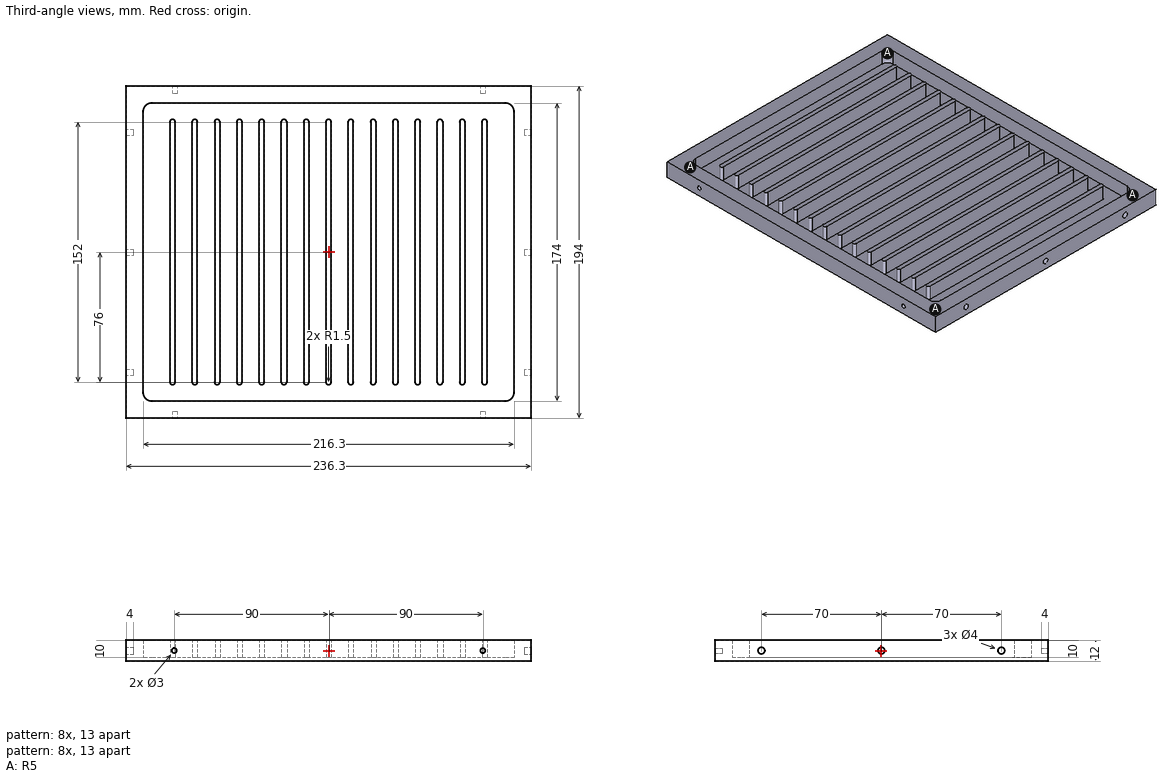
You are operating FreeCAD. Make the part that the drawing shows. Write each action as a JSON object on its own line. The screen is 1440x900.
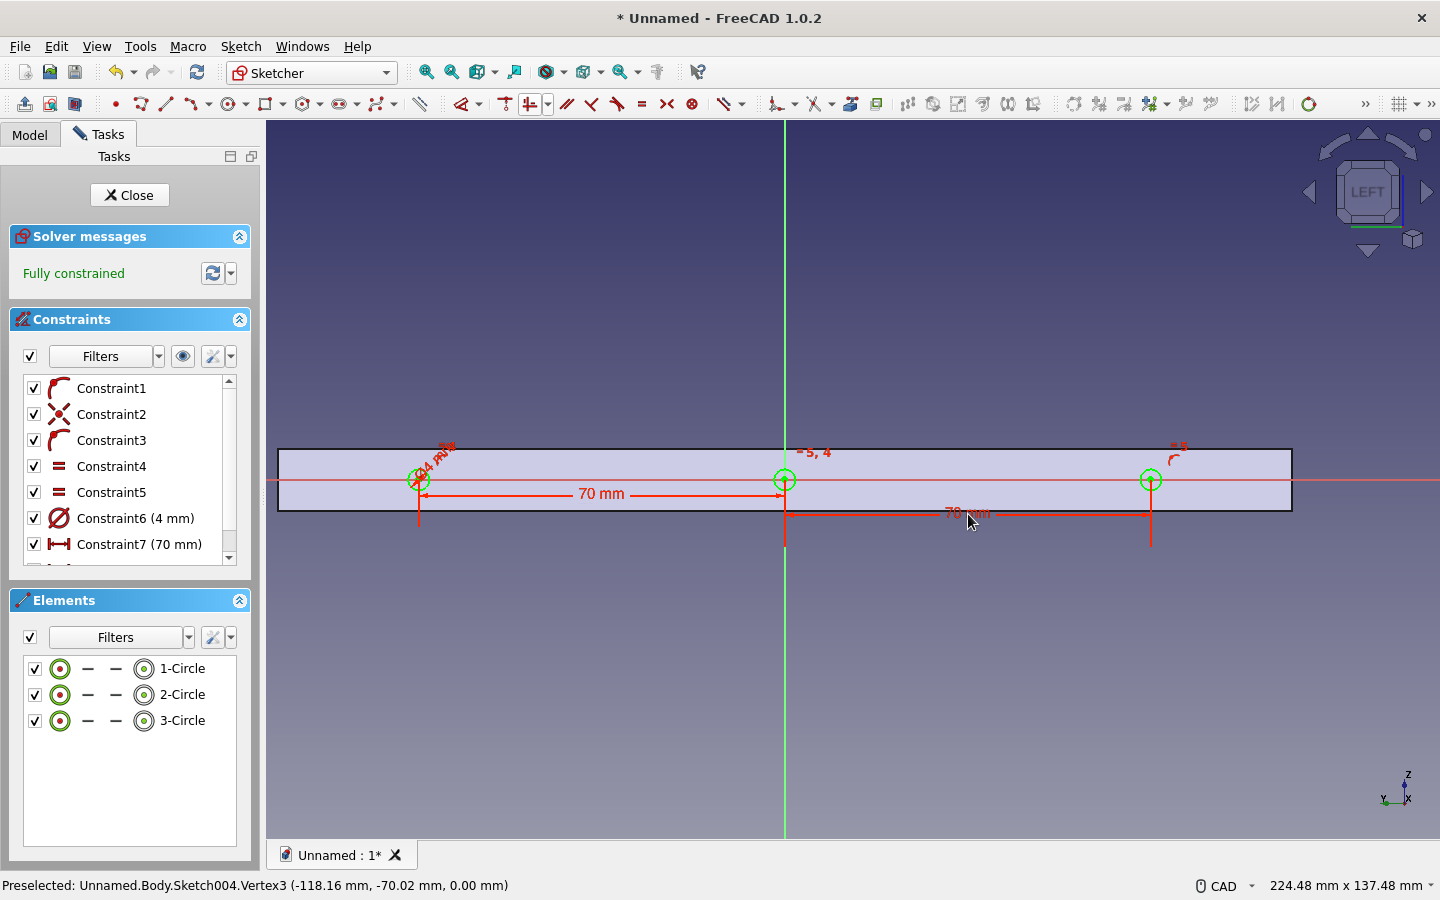
{"action": "left_click", "coordinate": [130, 195]}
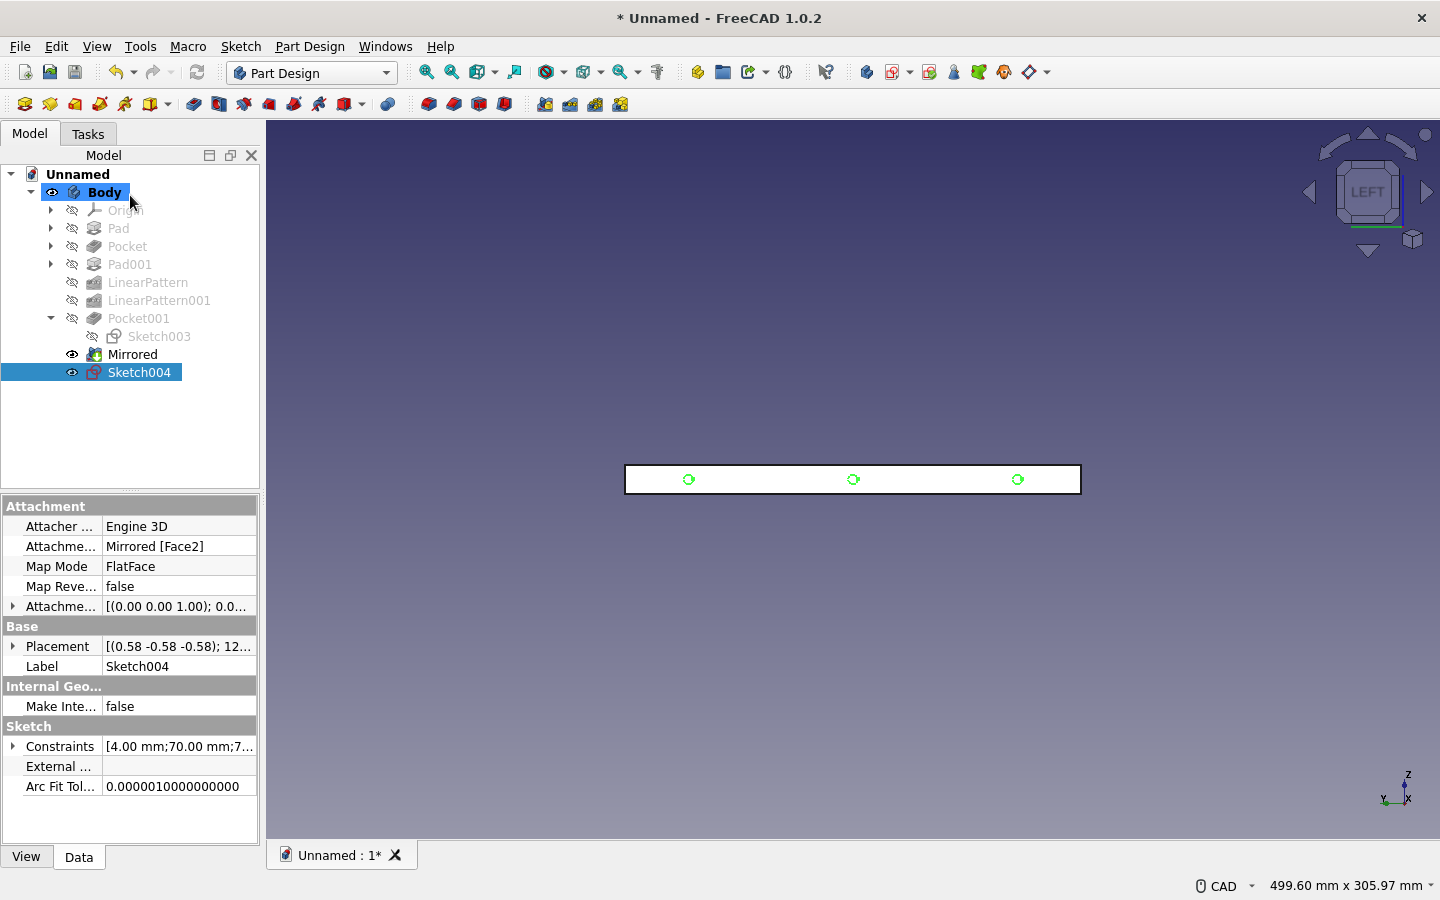
{"action": "left_click", "coordinate": [194, 104]}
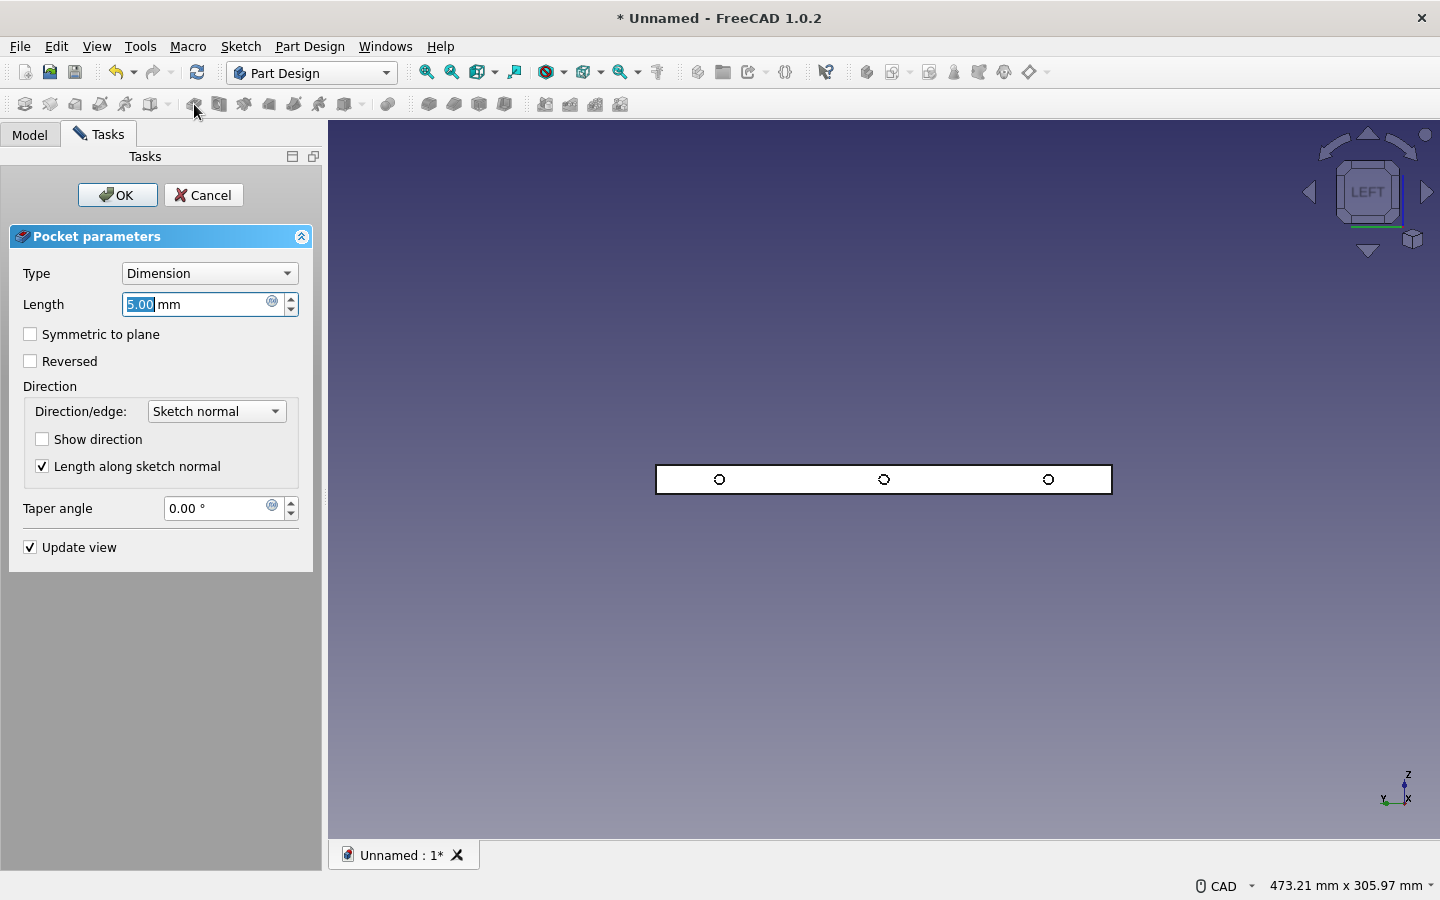
{"action": "type", "text": "4"}
{"action": "key", "text": "Tab"}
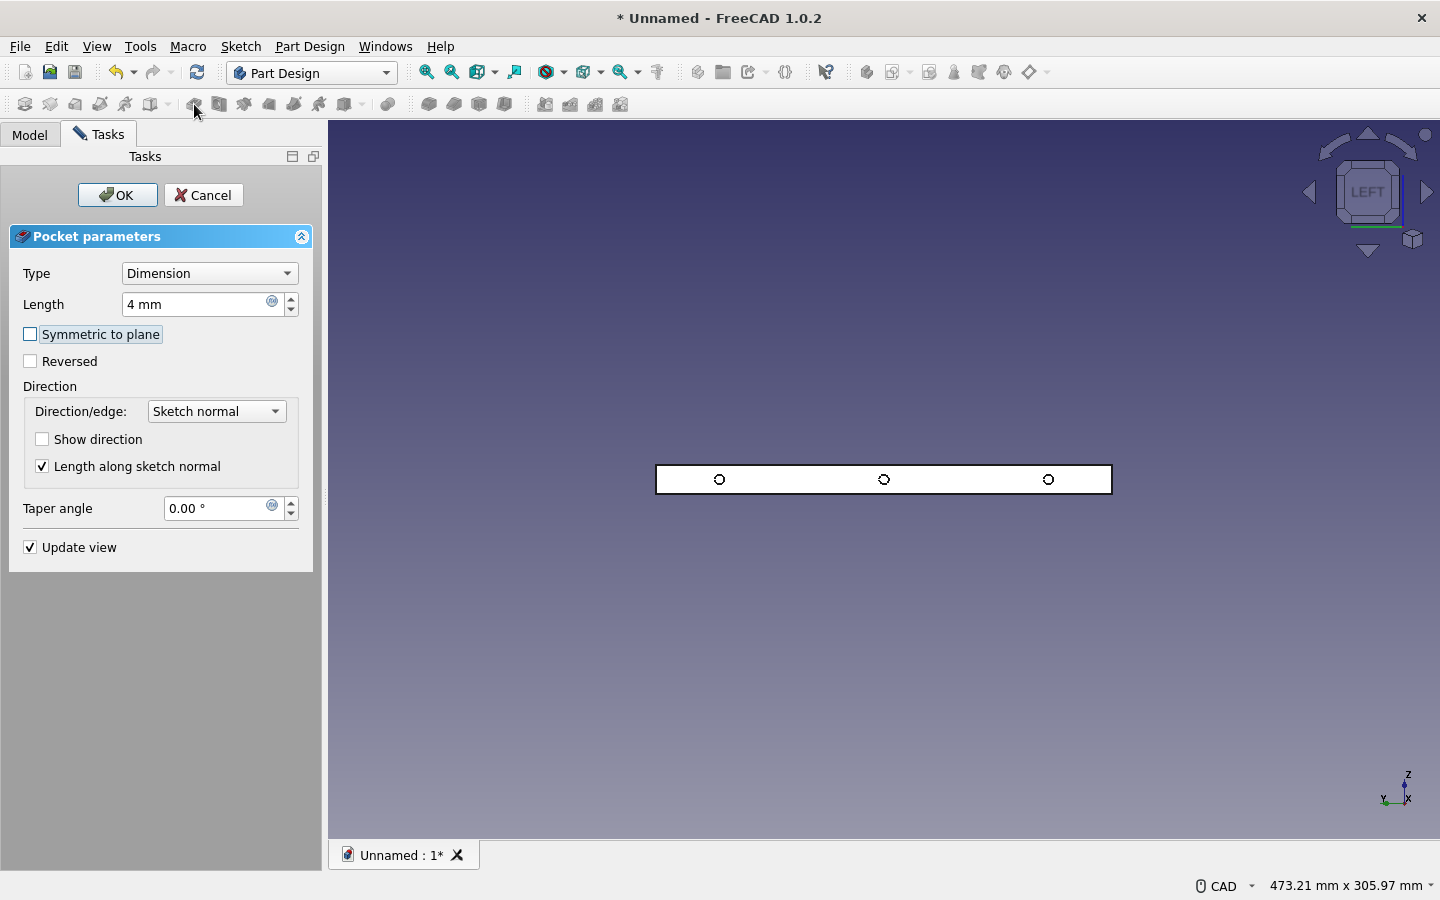
{"action": "left_click", "coordinate": [118, 195]}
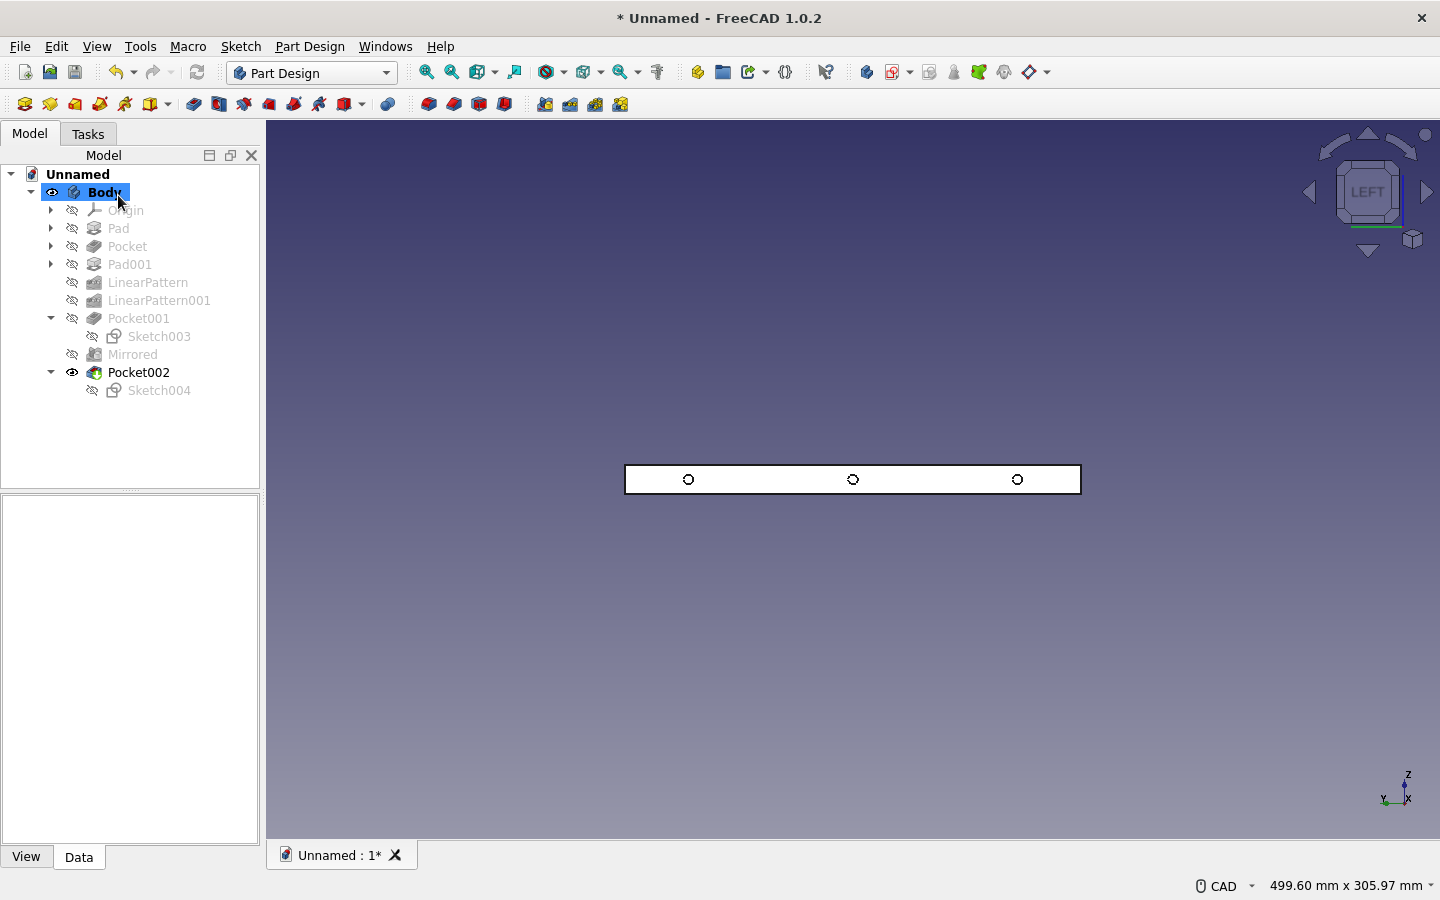
{"action": "left_click", "coordinate": [427, 72]}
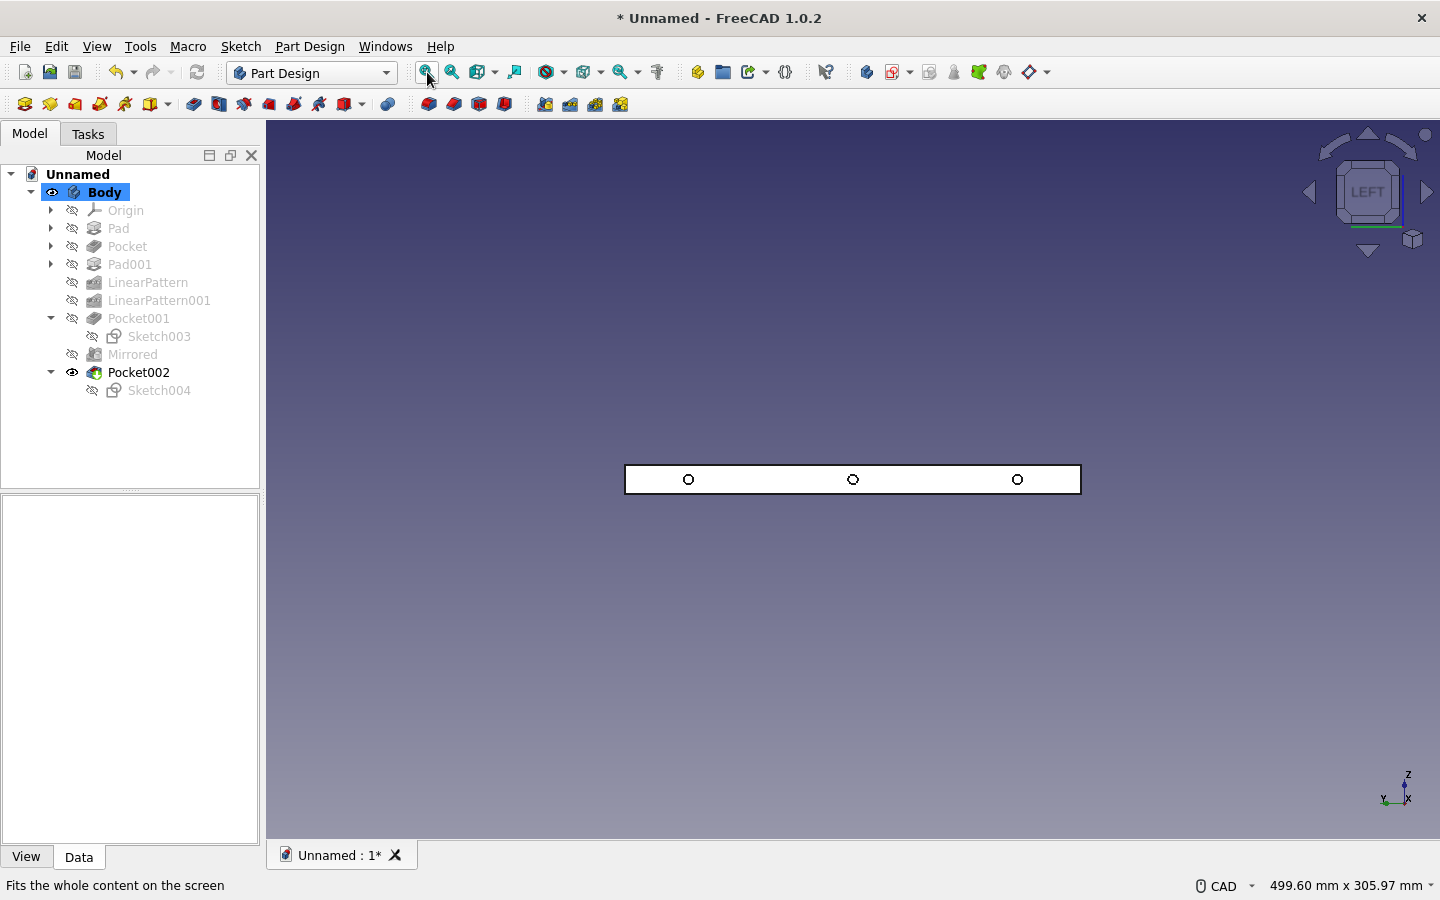
{"action": "left_click", "coordinate": [117, 372]}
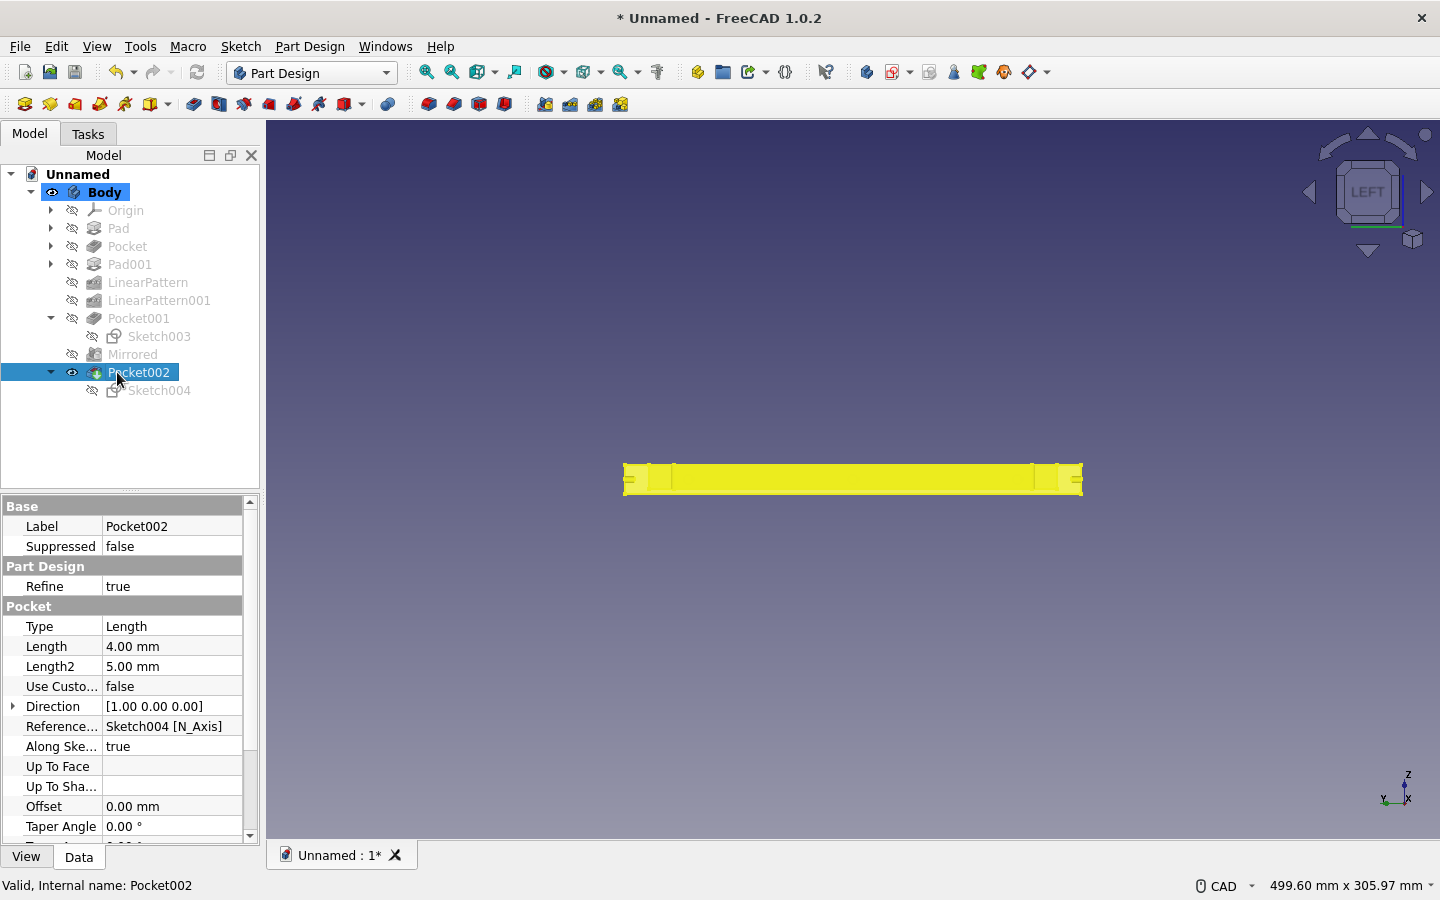
{"action": "left_click", "coordinate": [545, 104]}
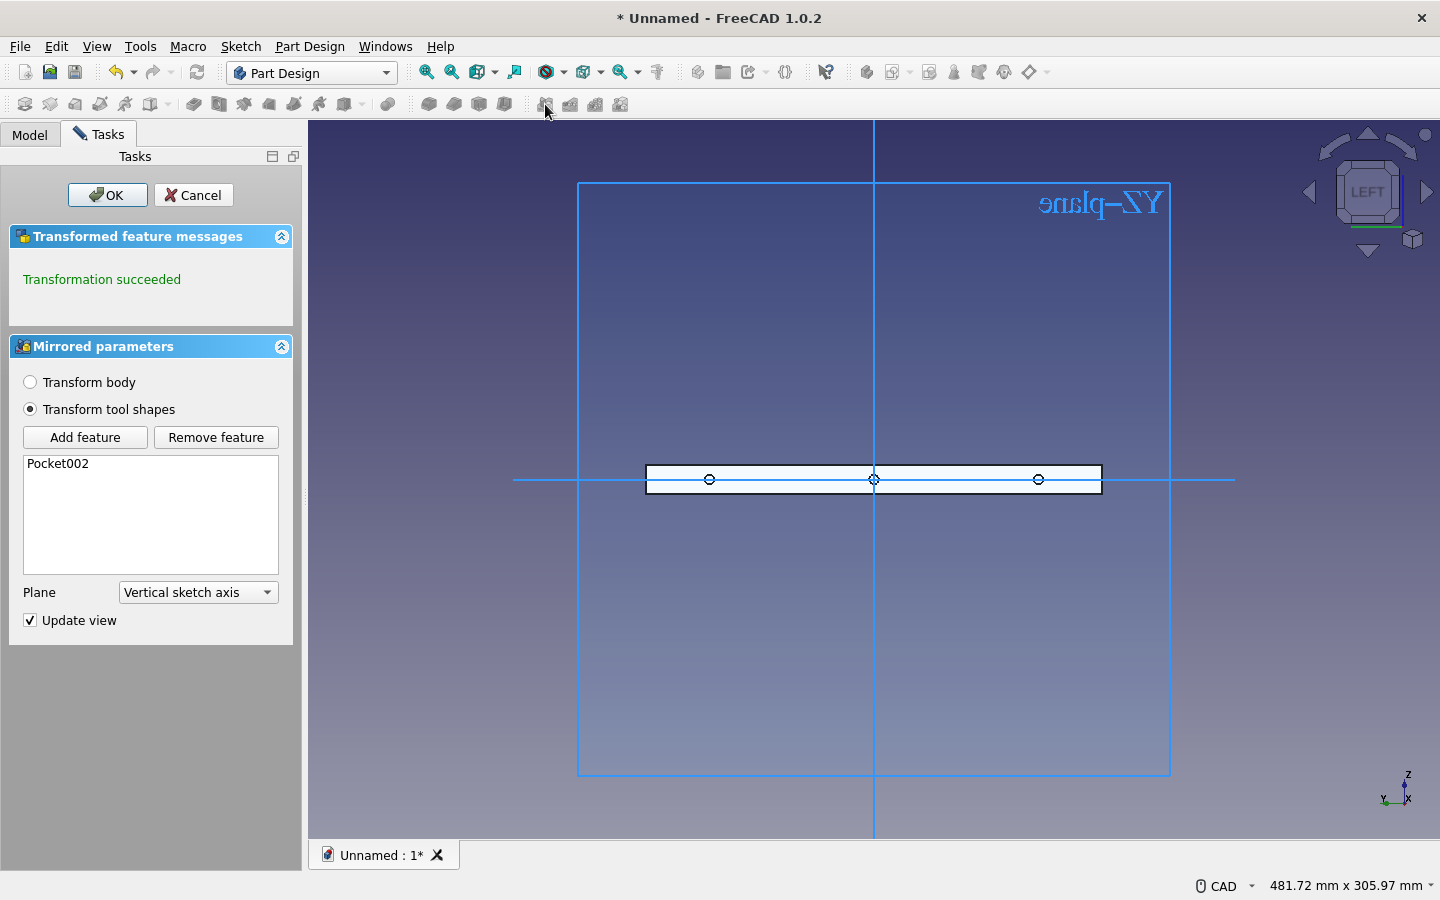
{"action": "left_click", "coordinate": [199, 592]}